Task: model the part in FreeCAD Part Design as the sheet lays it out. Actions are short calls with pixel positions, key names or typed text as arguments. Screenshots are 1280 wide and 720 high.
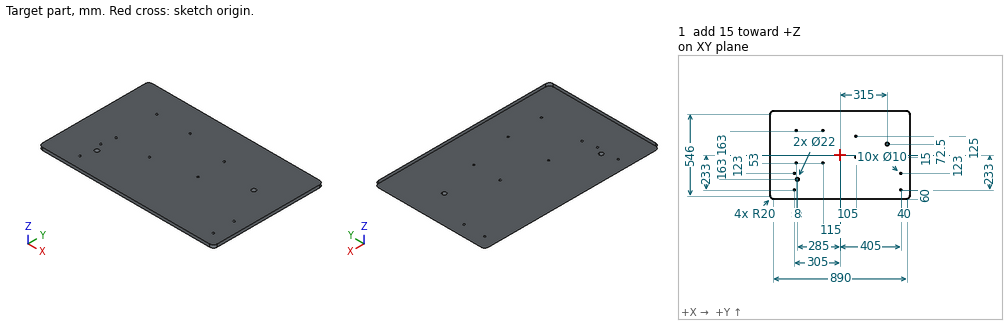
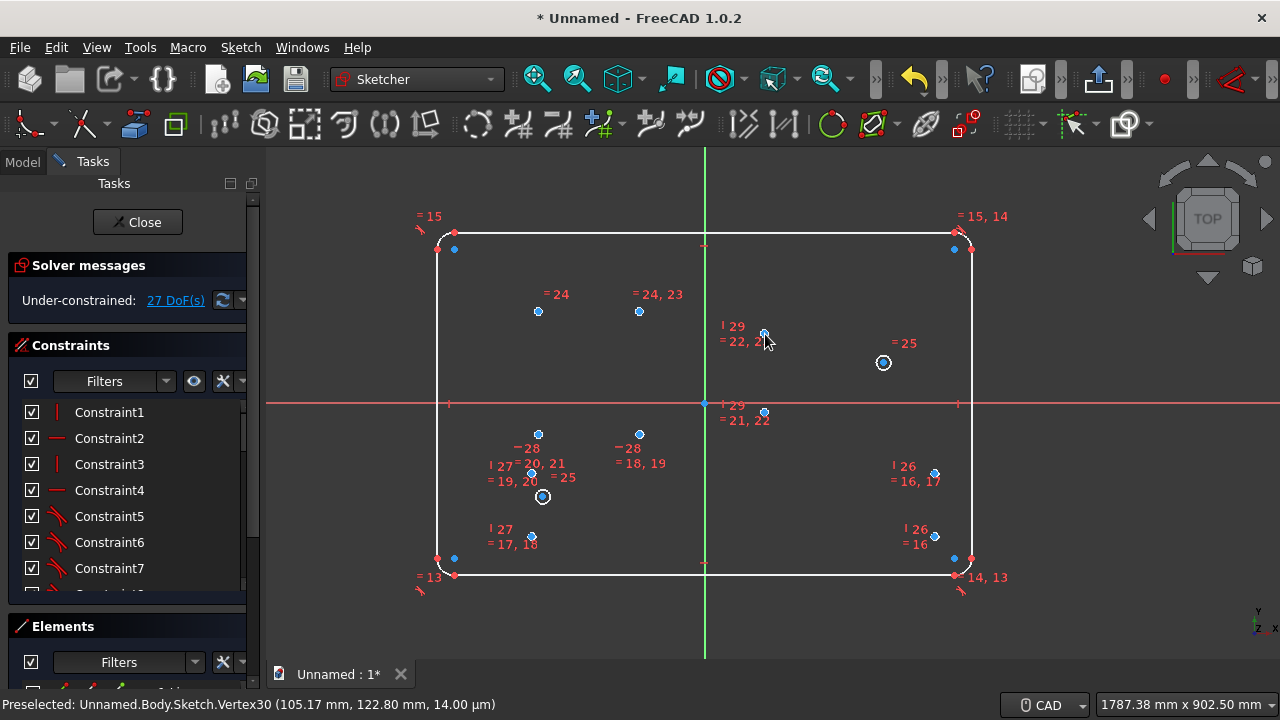
click(640, 435)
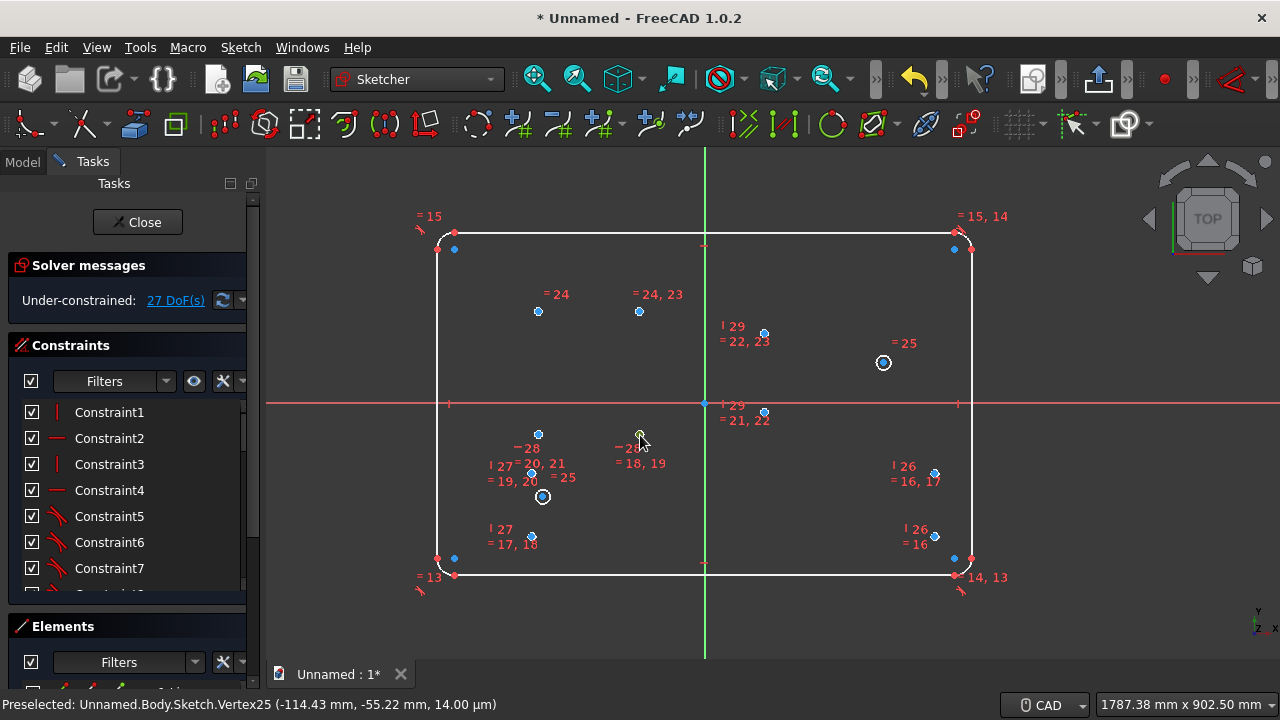
click(639, 312)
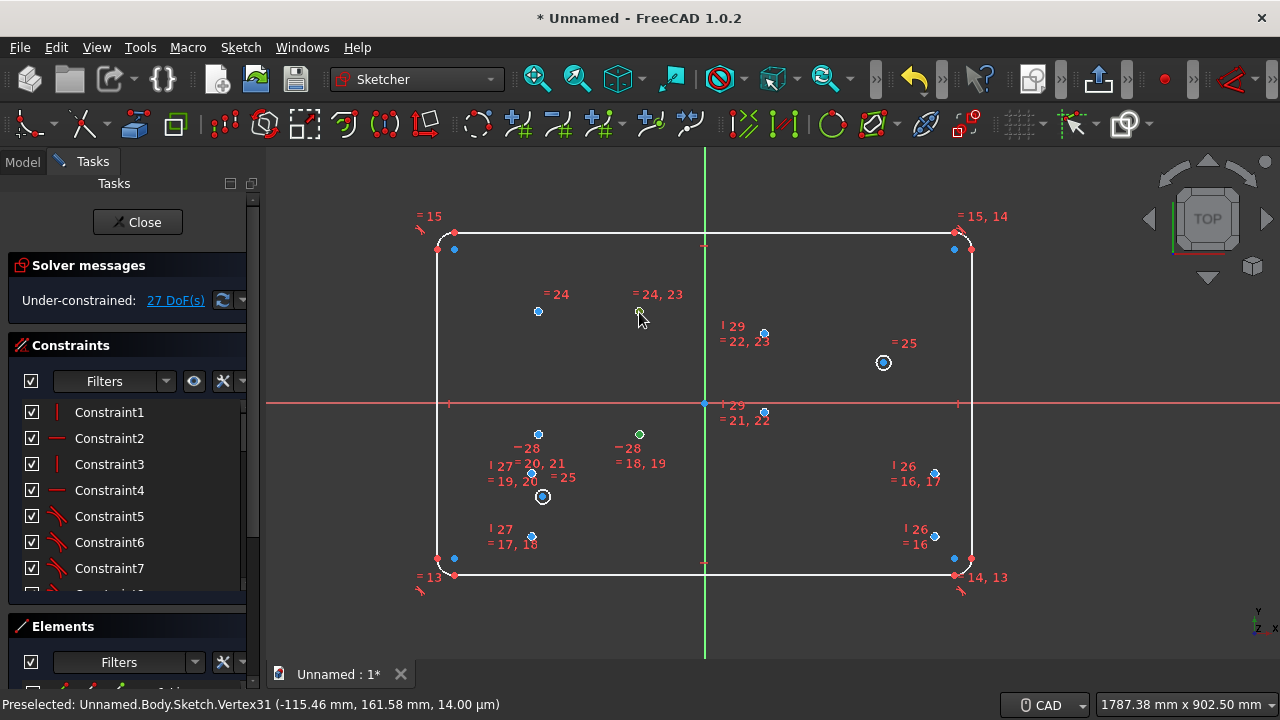
key(v)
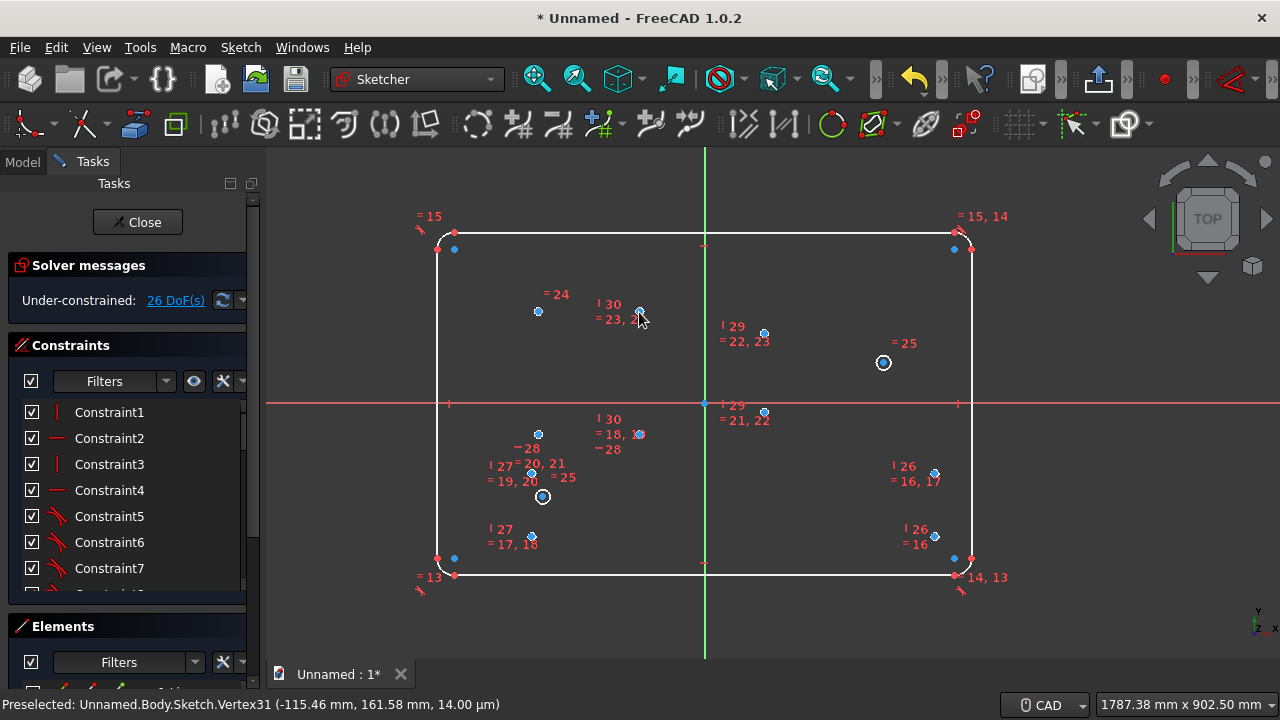
click(539, 435)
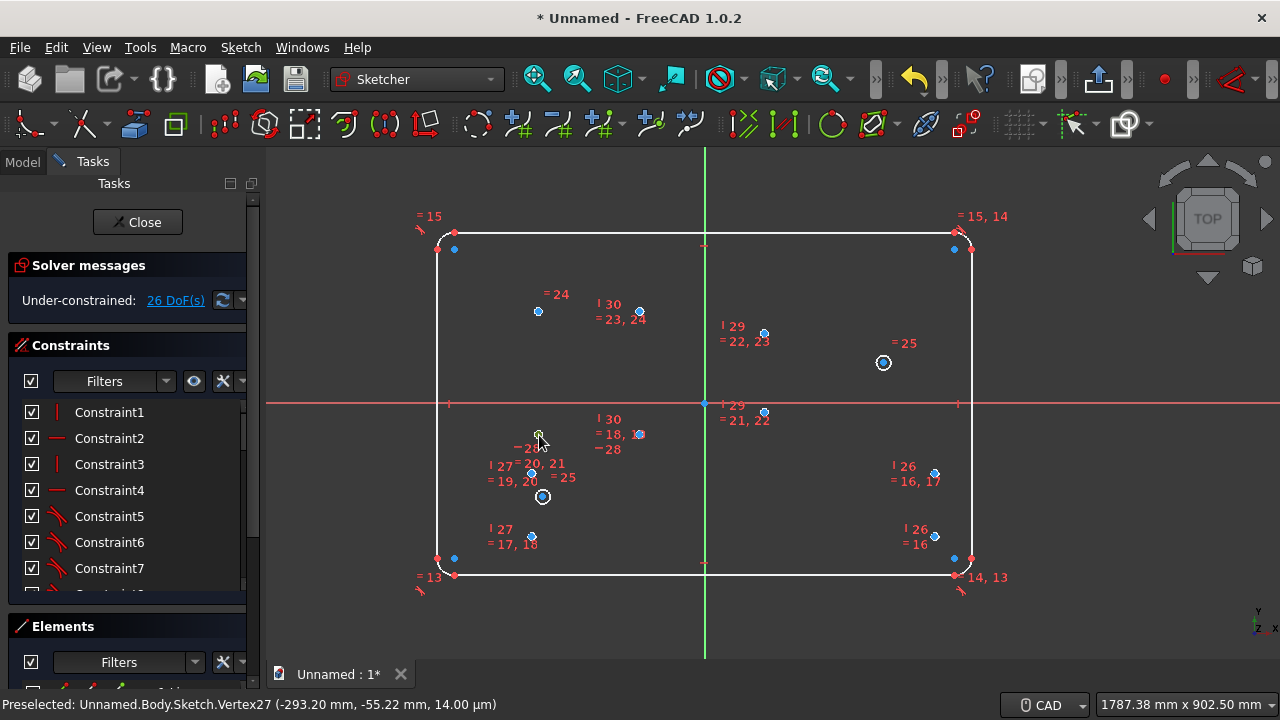
click(538, 312)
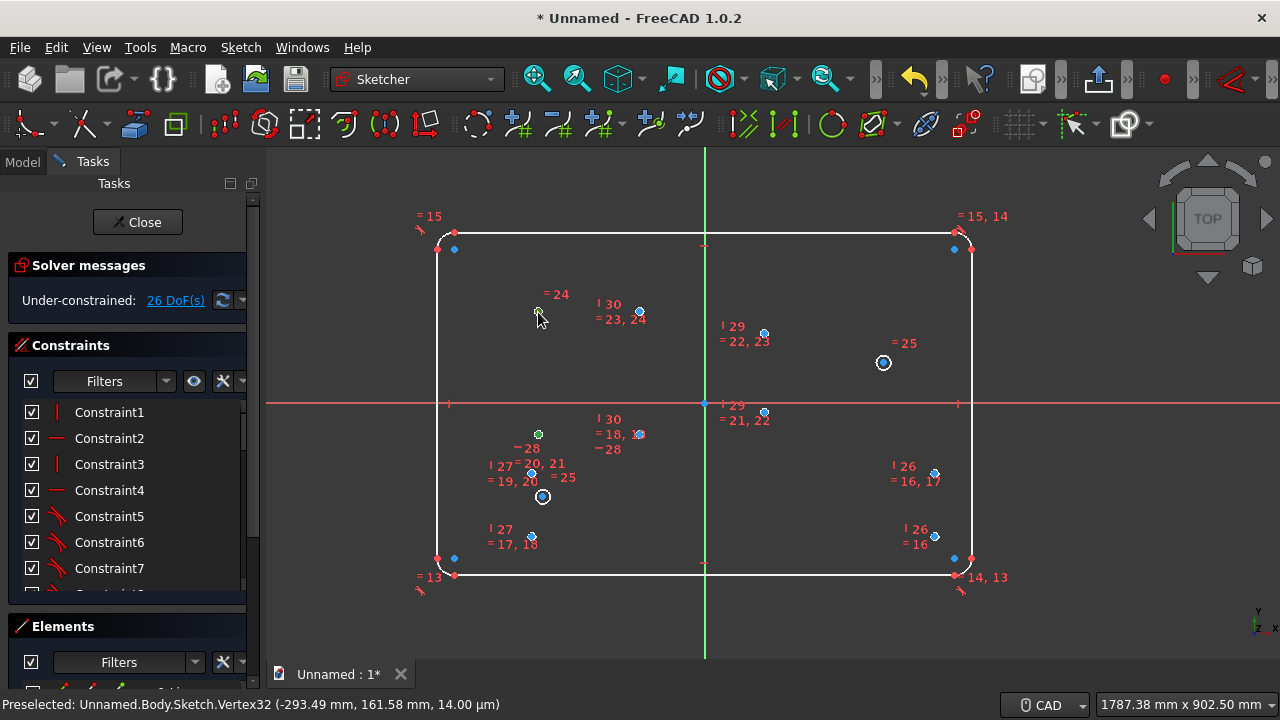
key(v)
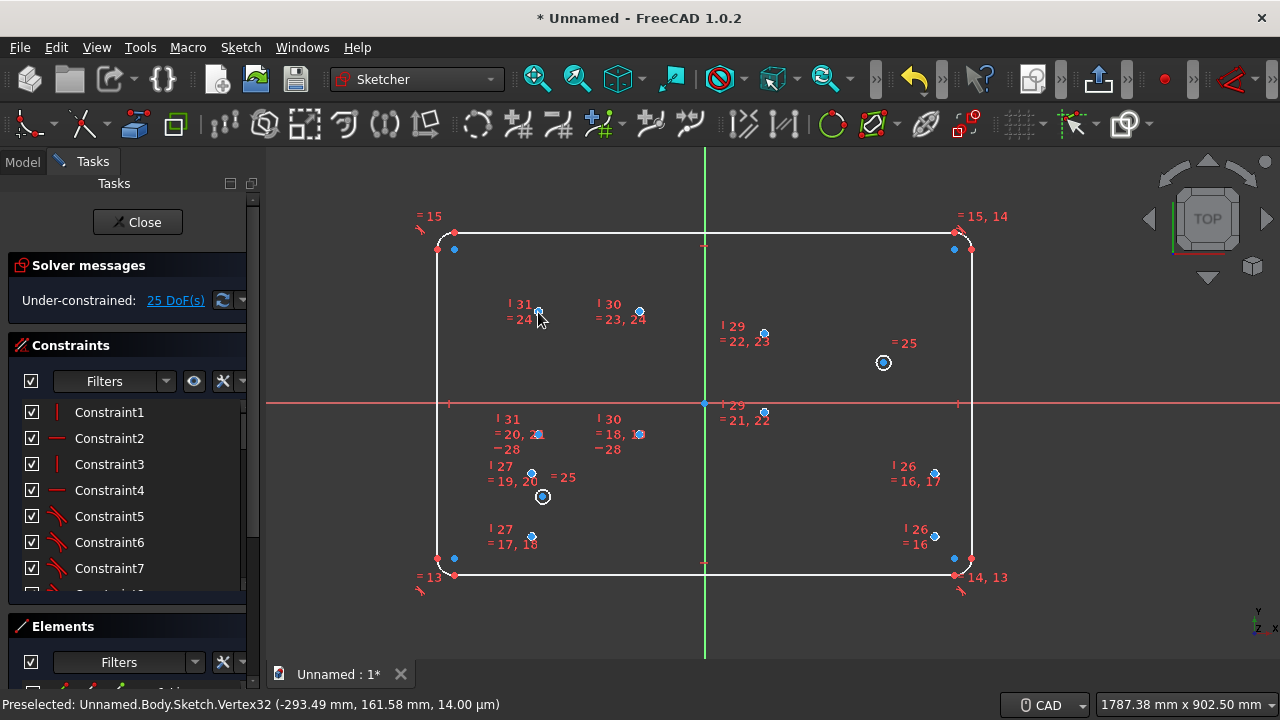
scroll(640, 312, up, 4)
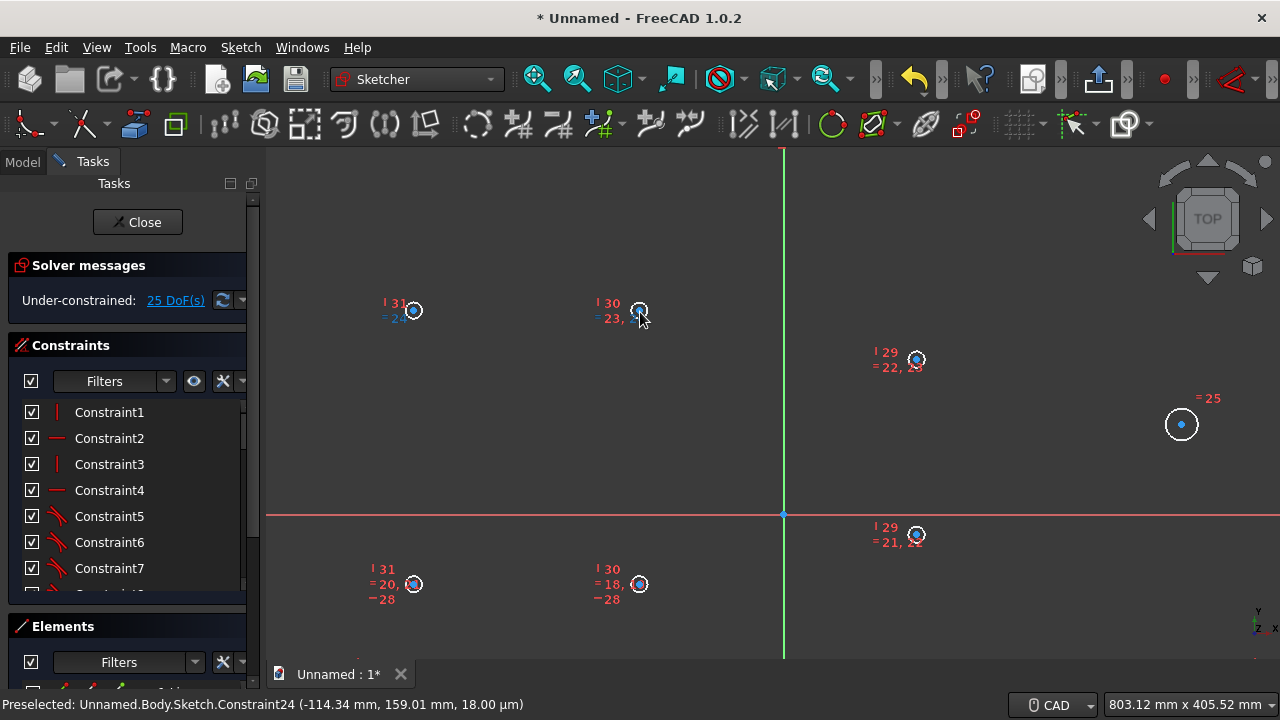
scroll(639, 311, up, 4)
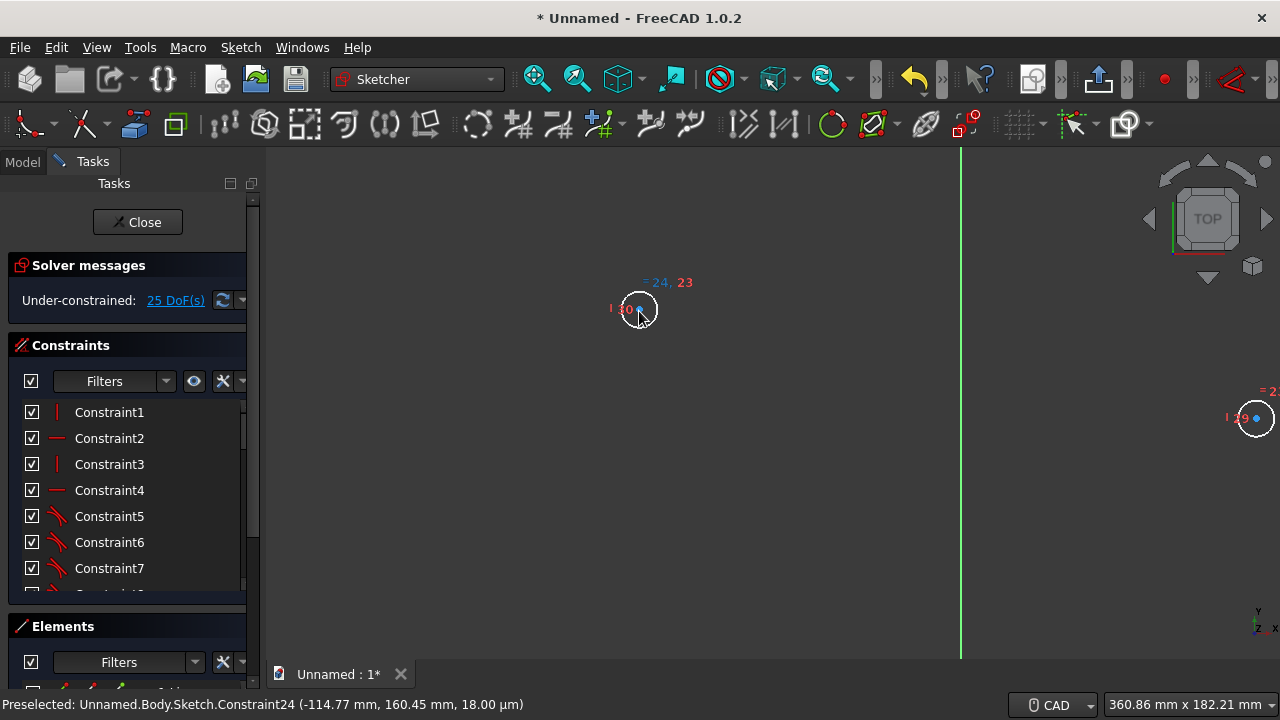
click(639, 310)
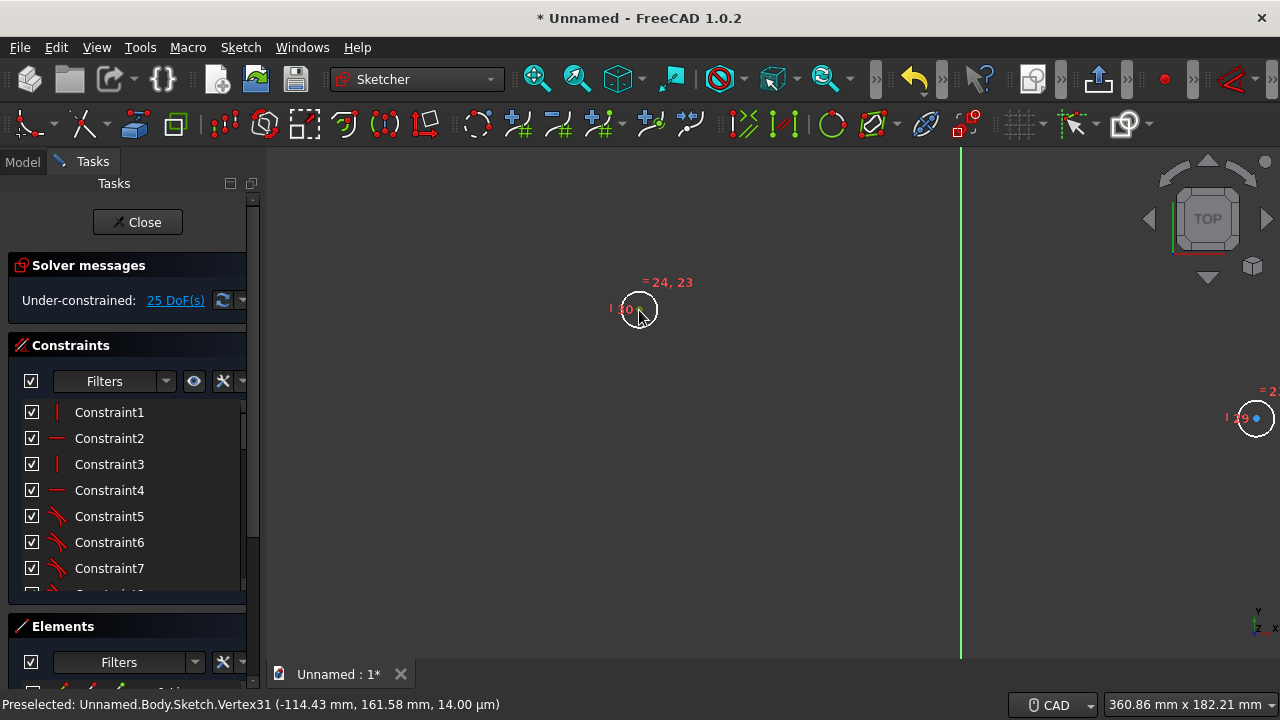
scroll(640, 312, down, 8)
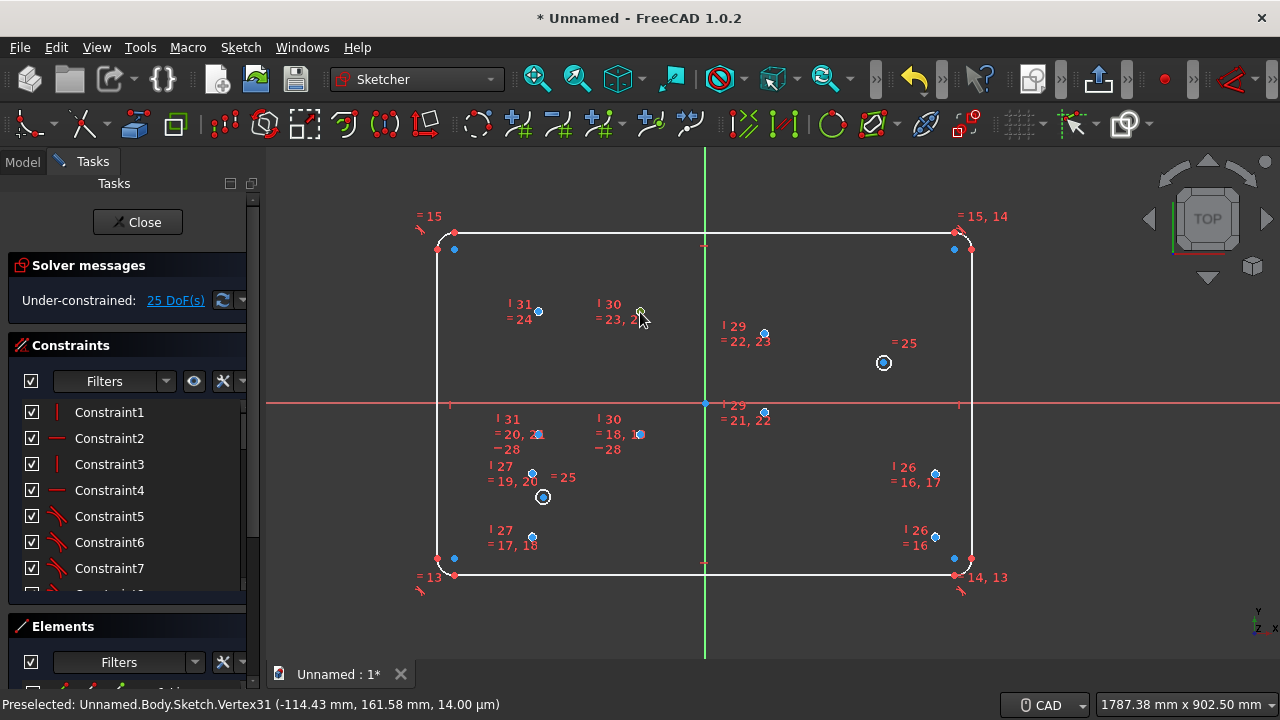
click(539, 312)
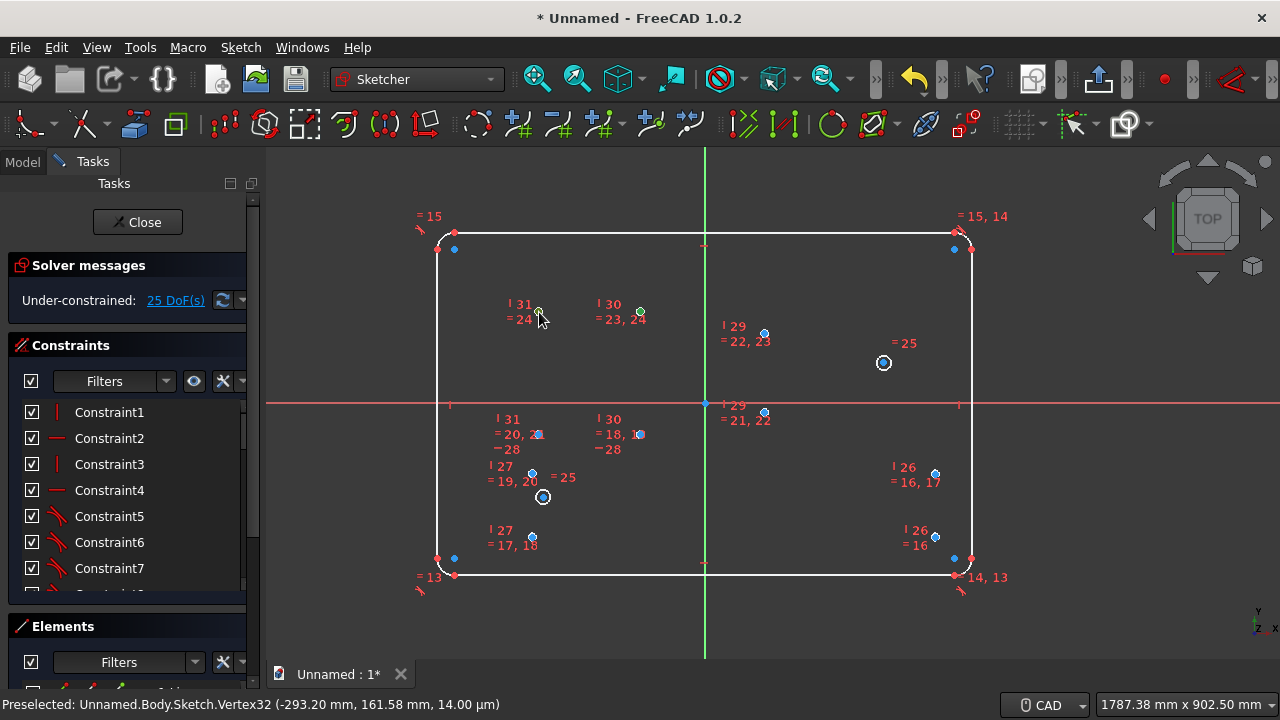
key(h)